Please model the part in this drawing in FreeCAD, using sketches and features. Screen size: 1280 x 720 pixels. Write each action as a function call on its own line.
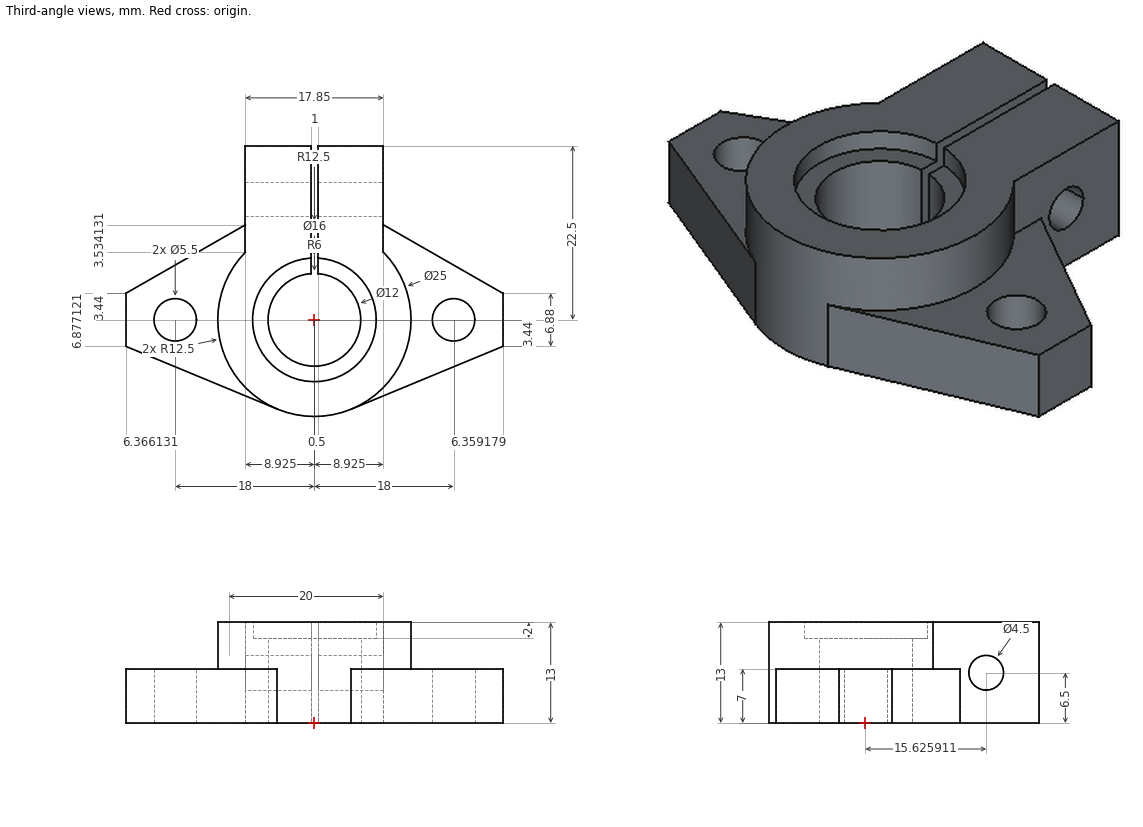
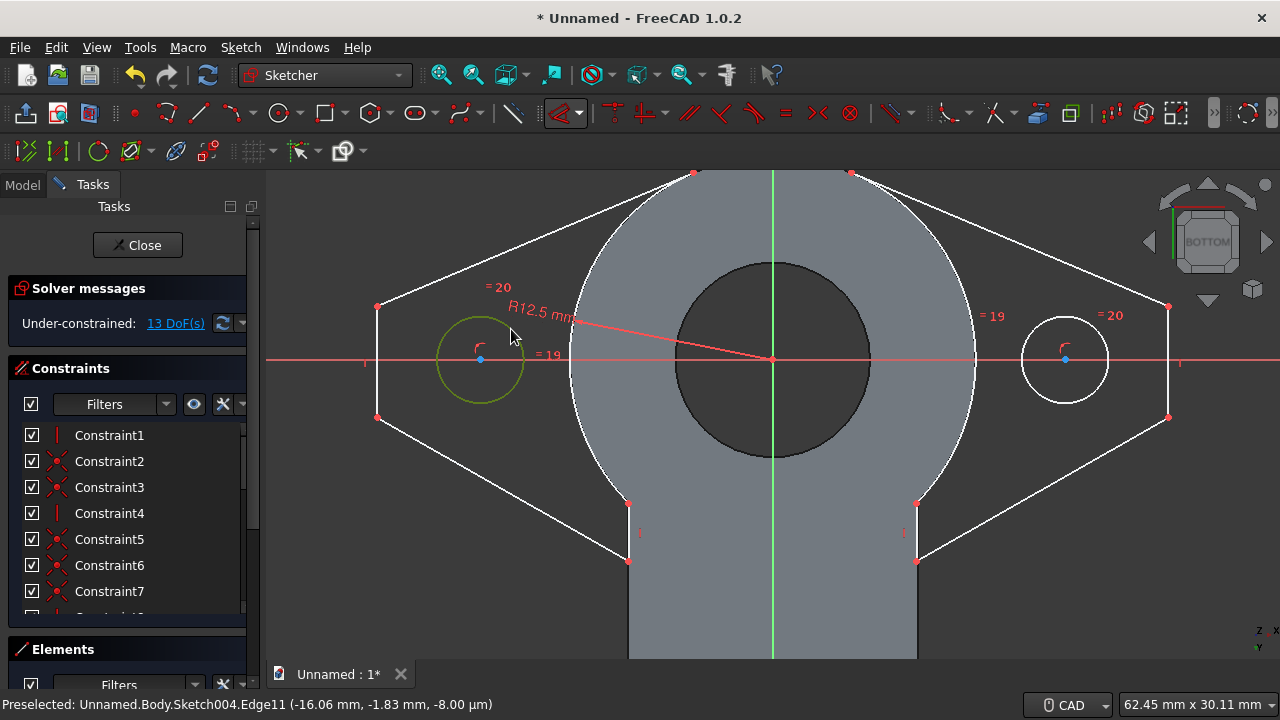
key(k)
key(o)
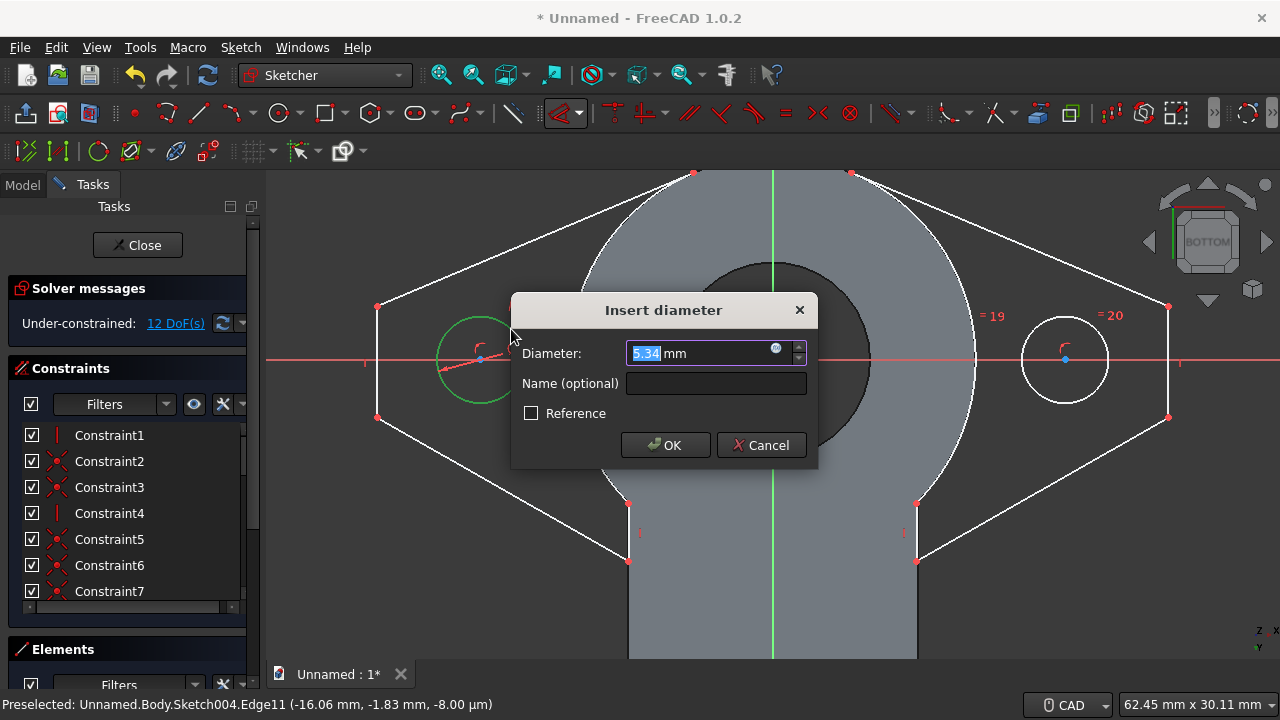
text(5.5)
key(Return)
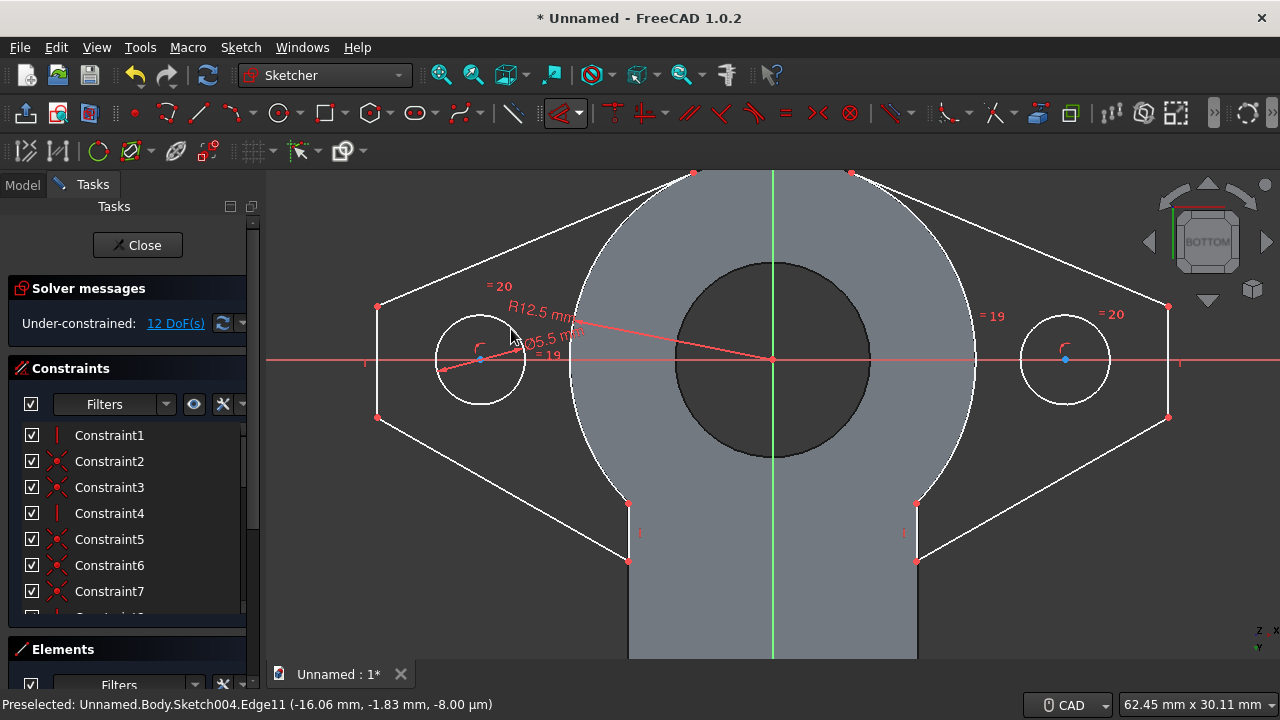
click(480, 360)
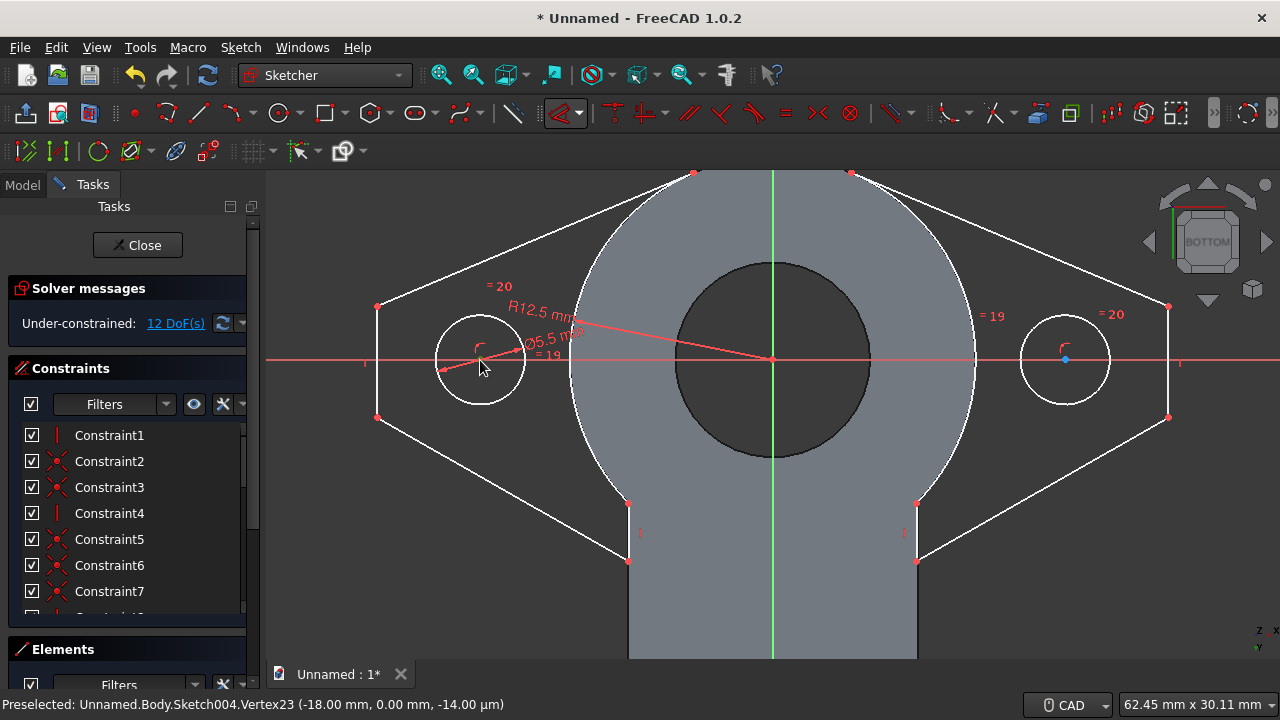
click(582, 114)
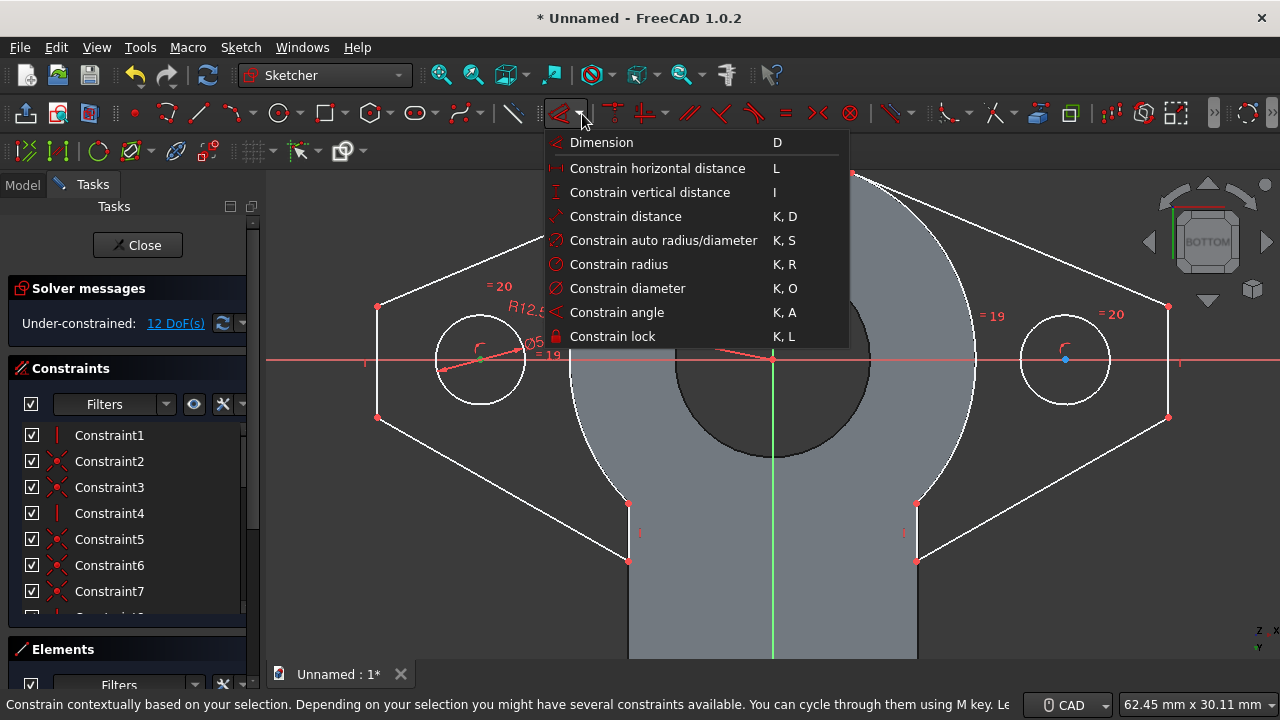
click(697, 168)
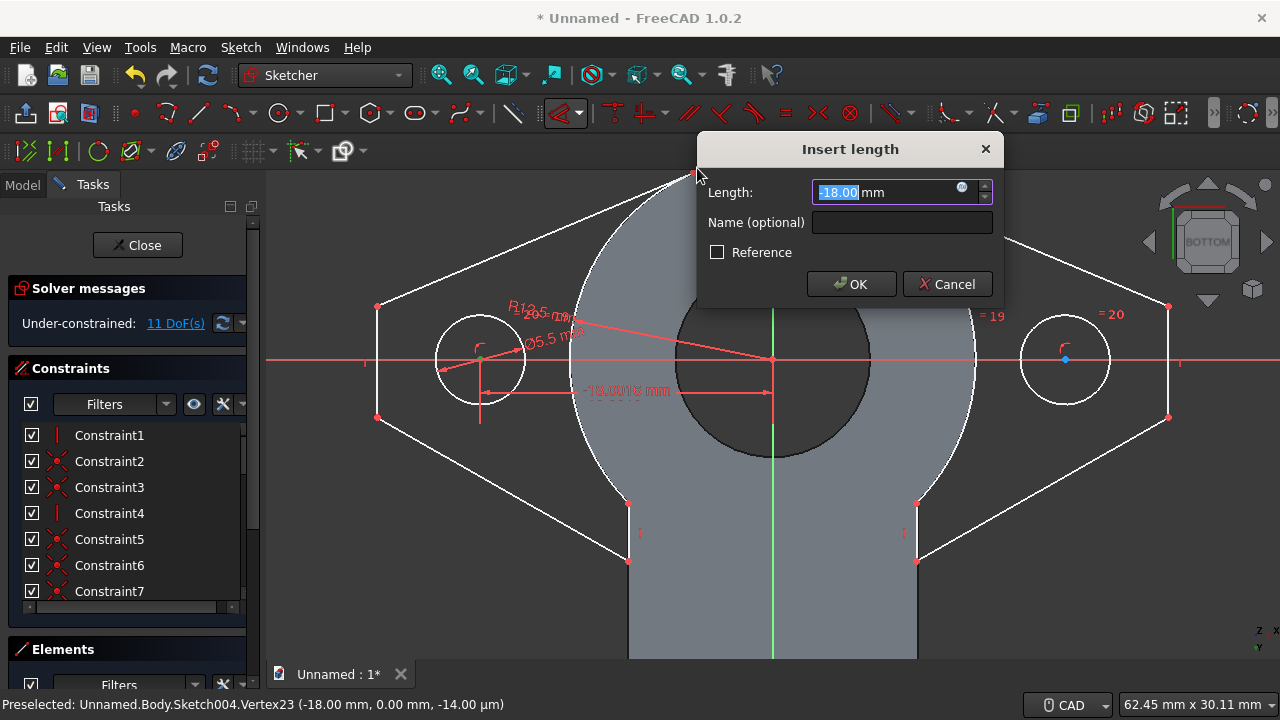
text(-18)
key(Return)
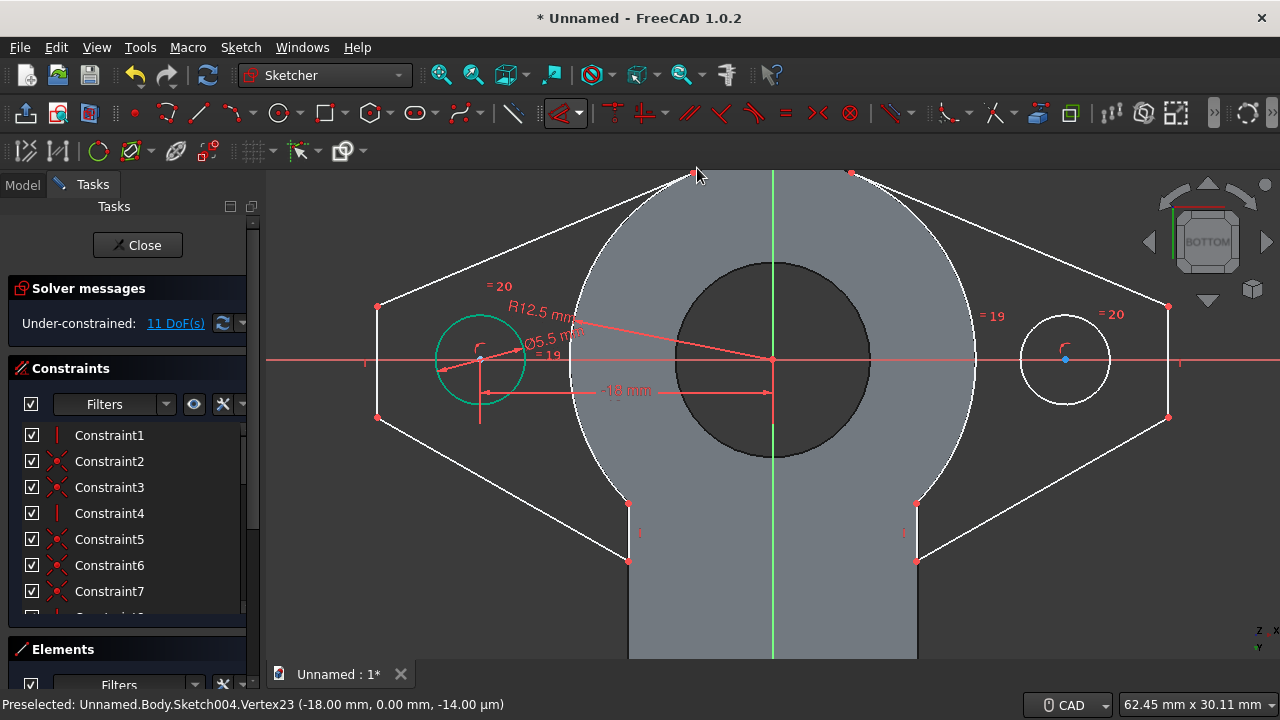
click(1065, 360)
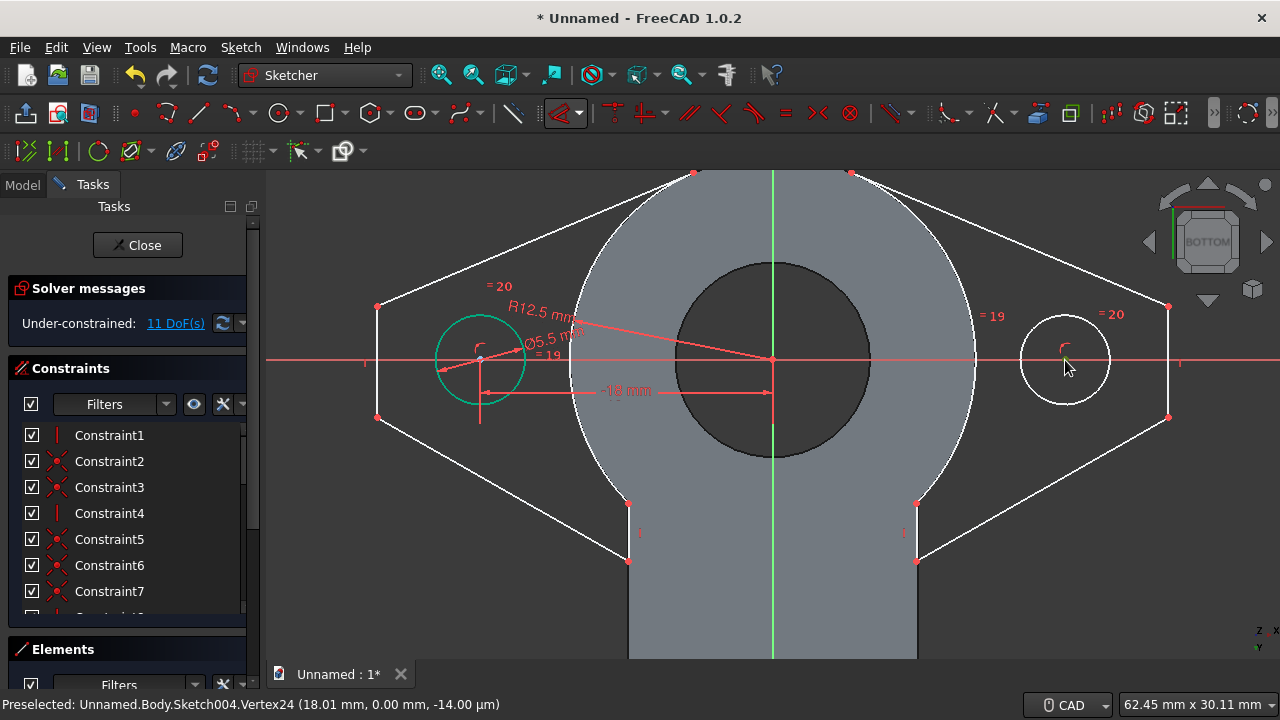
key(l)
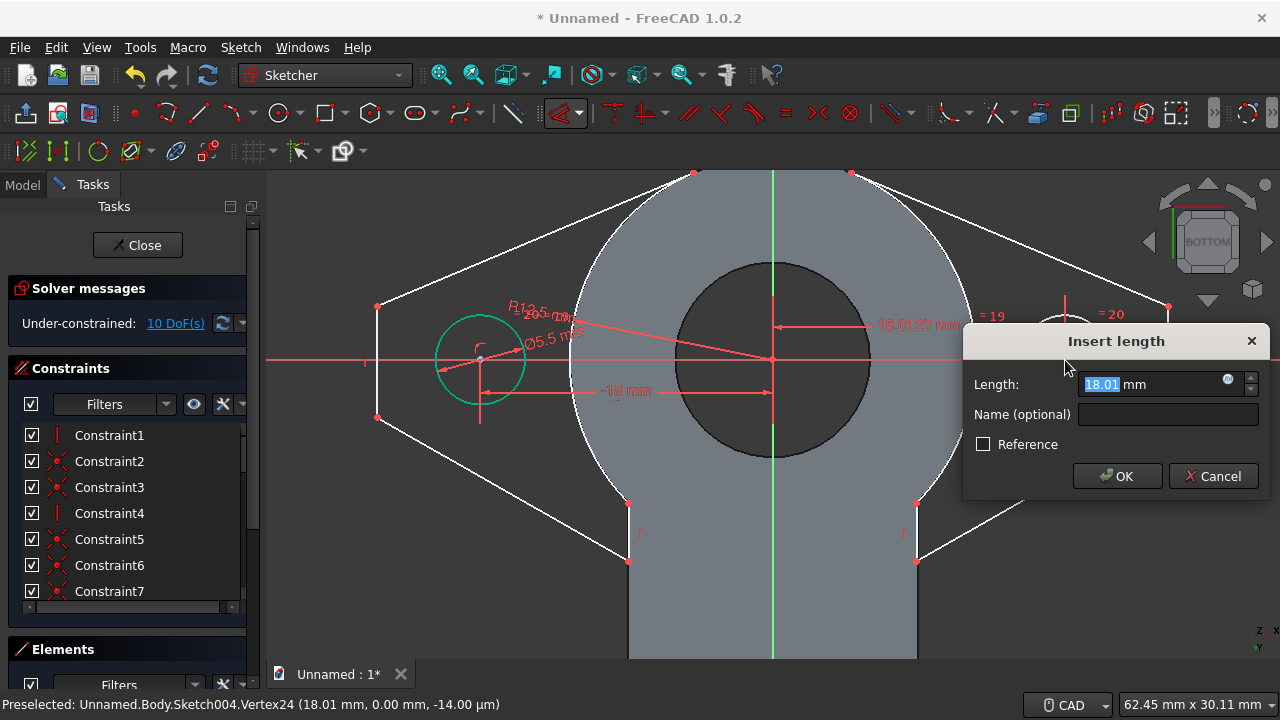
text(18)
key(Return)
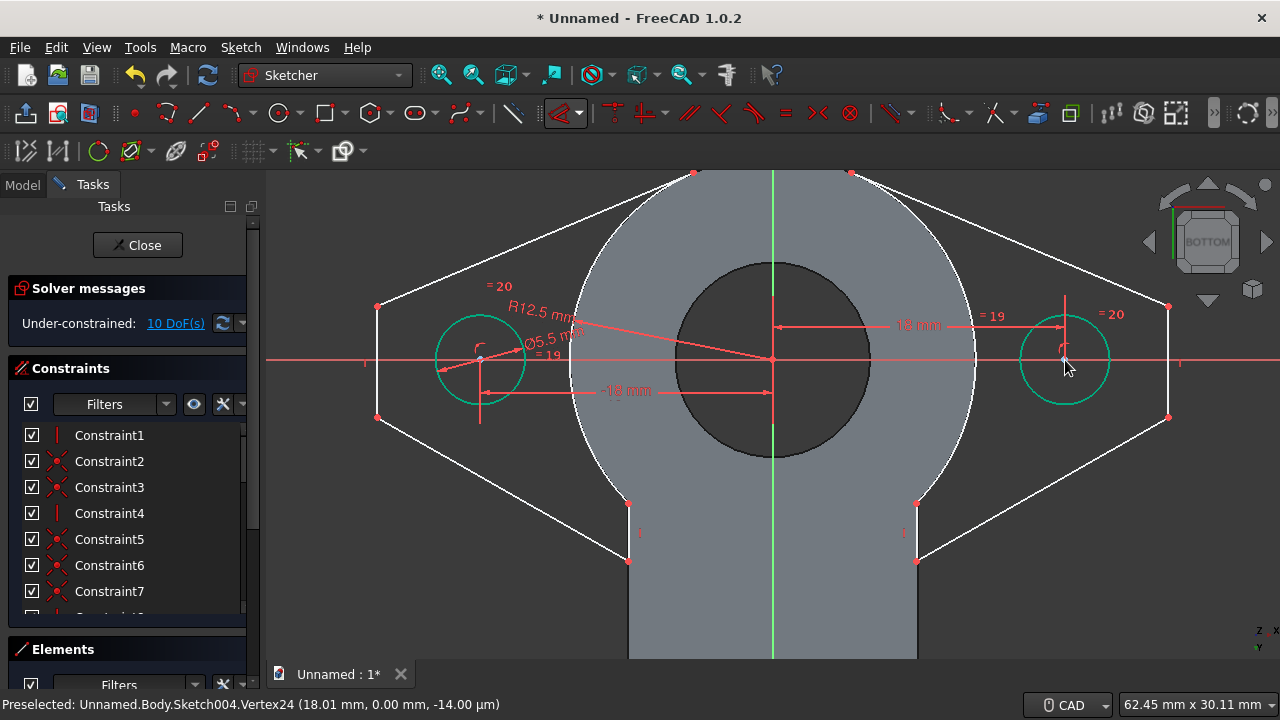
scroll(566, 513, down, 2)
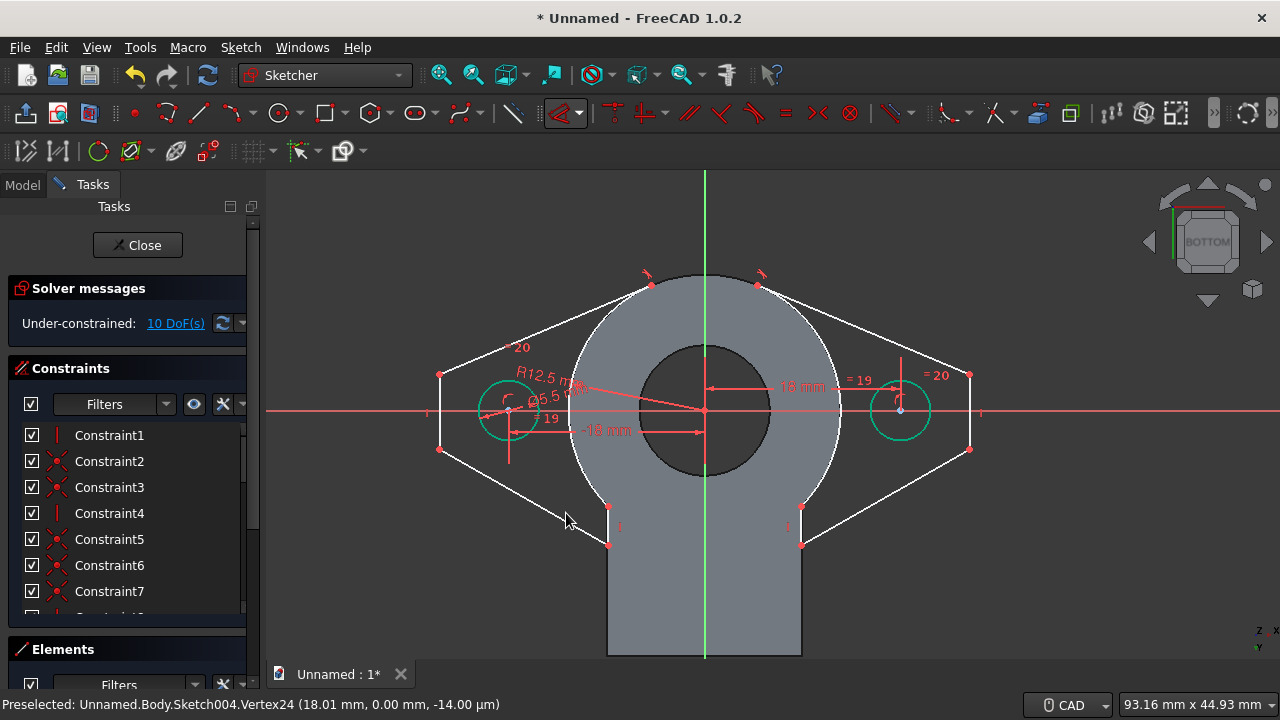
click(970, 397)